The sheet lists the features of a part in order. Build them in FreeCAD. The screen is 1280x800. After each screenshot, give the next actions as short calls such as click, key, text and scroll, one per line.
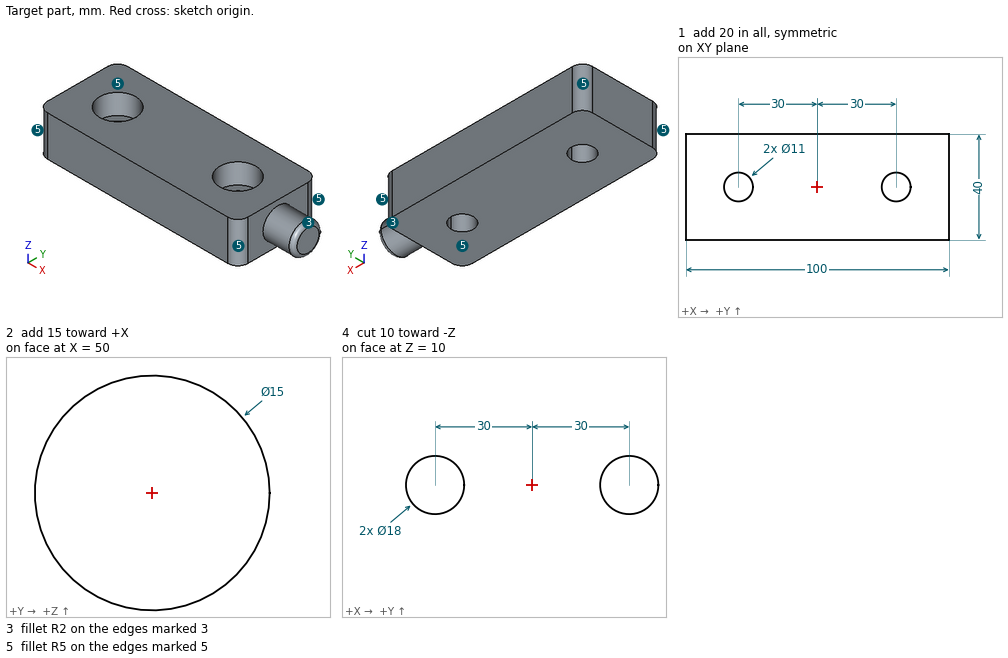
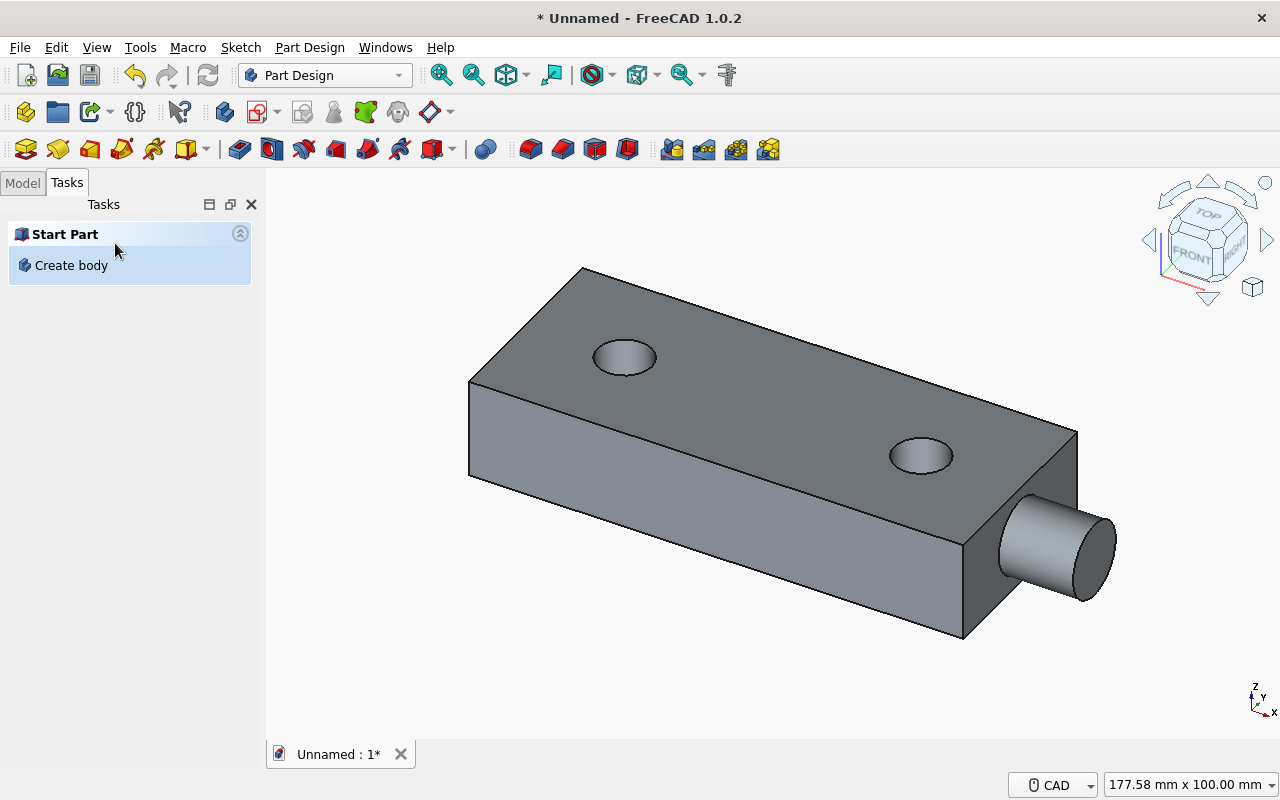
click(1073, 580)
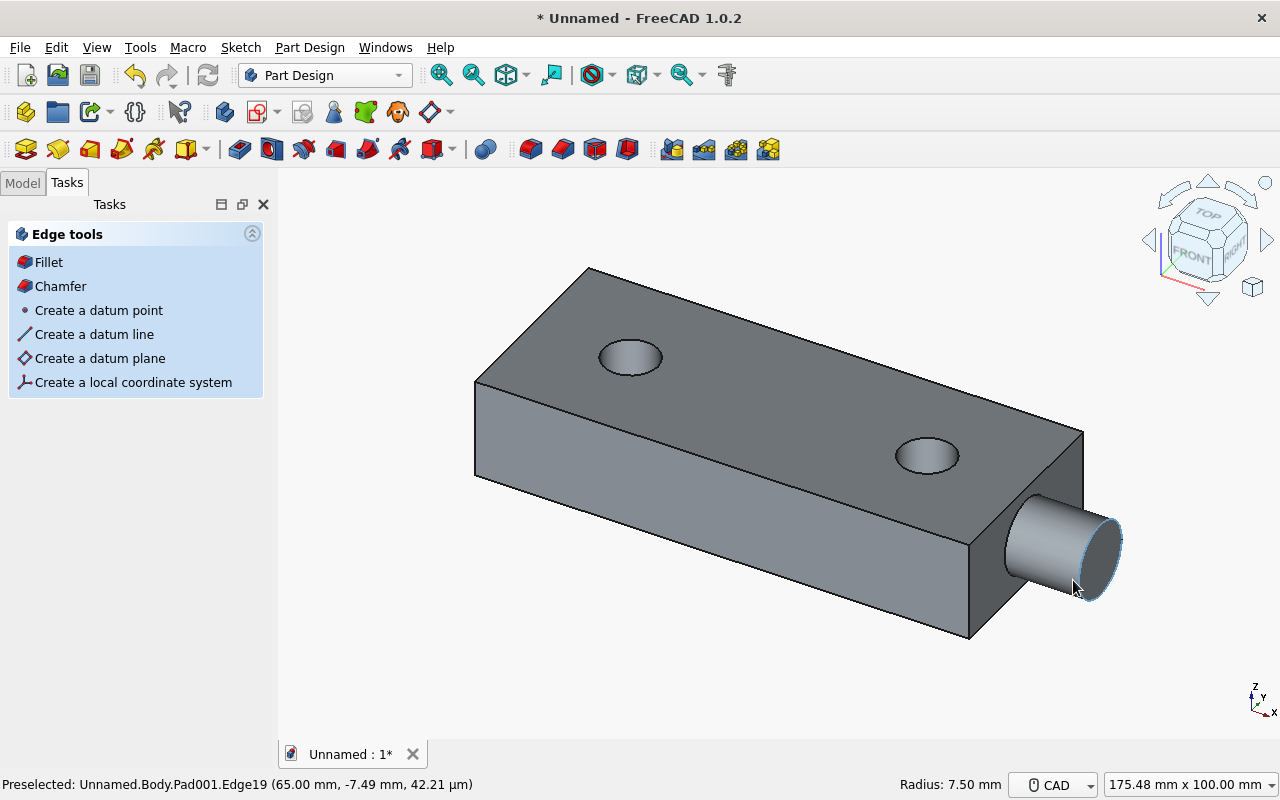
click(532, 150)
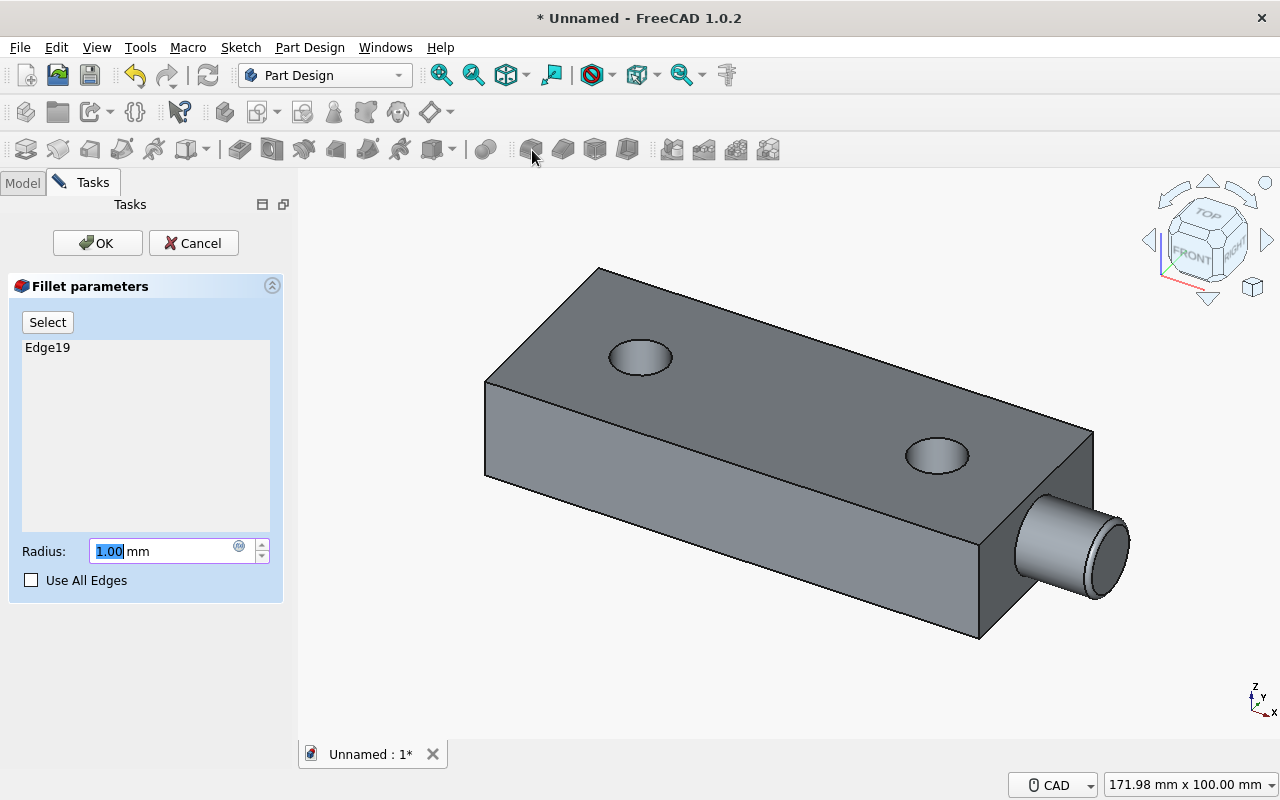
text(2)
key(Tab)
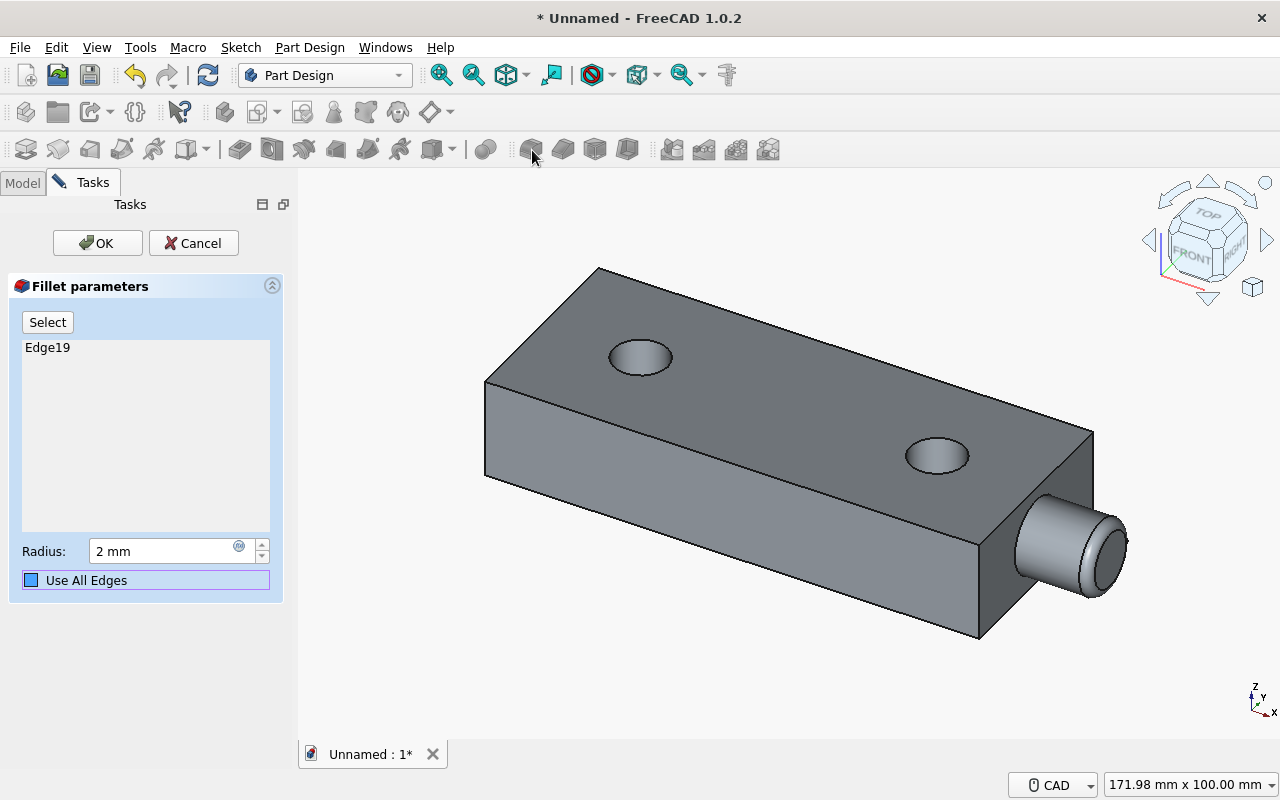
click(98, 243)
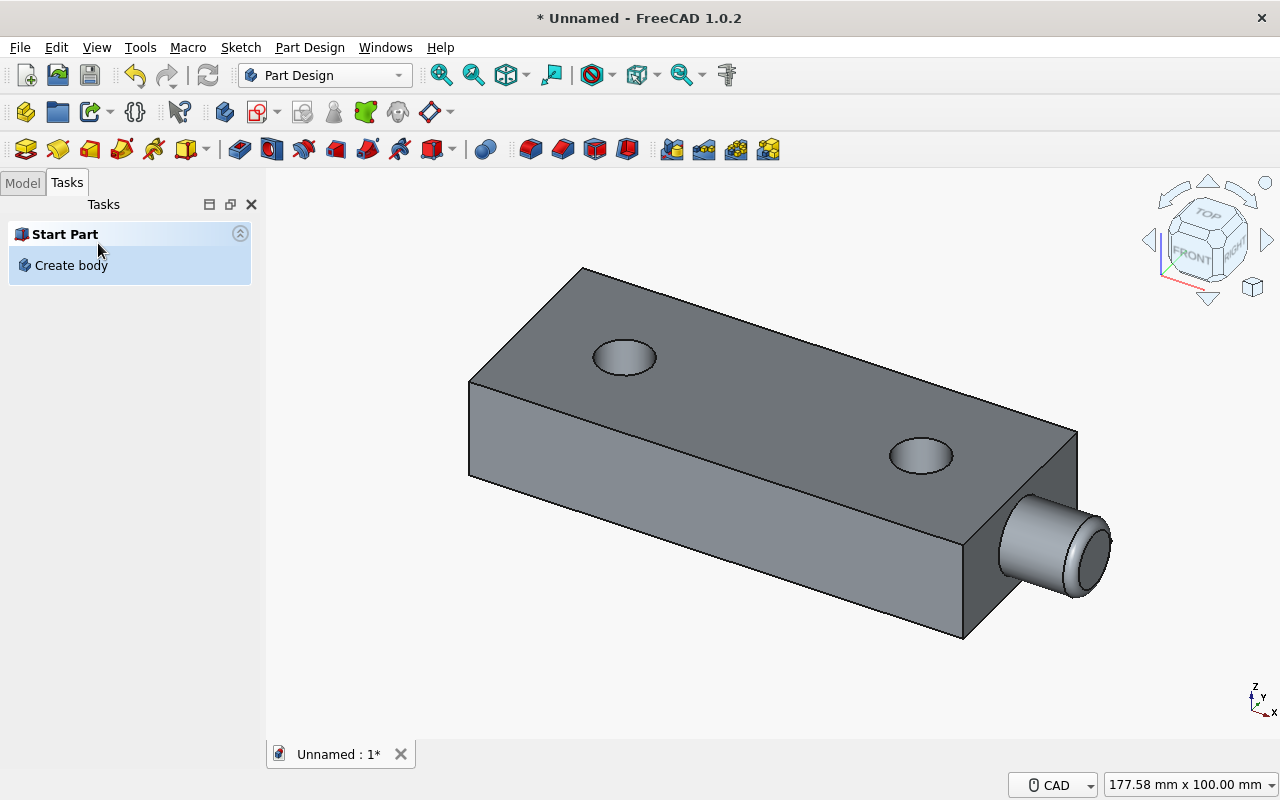
click(773, 406)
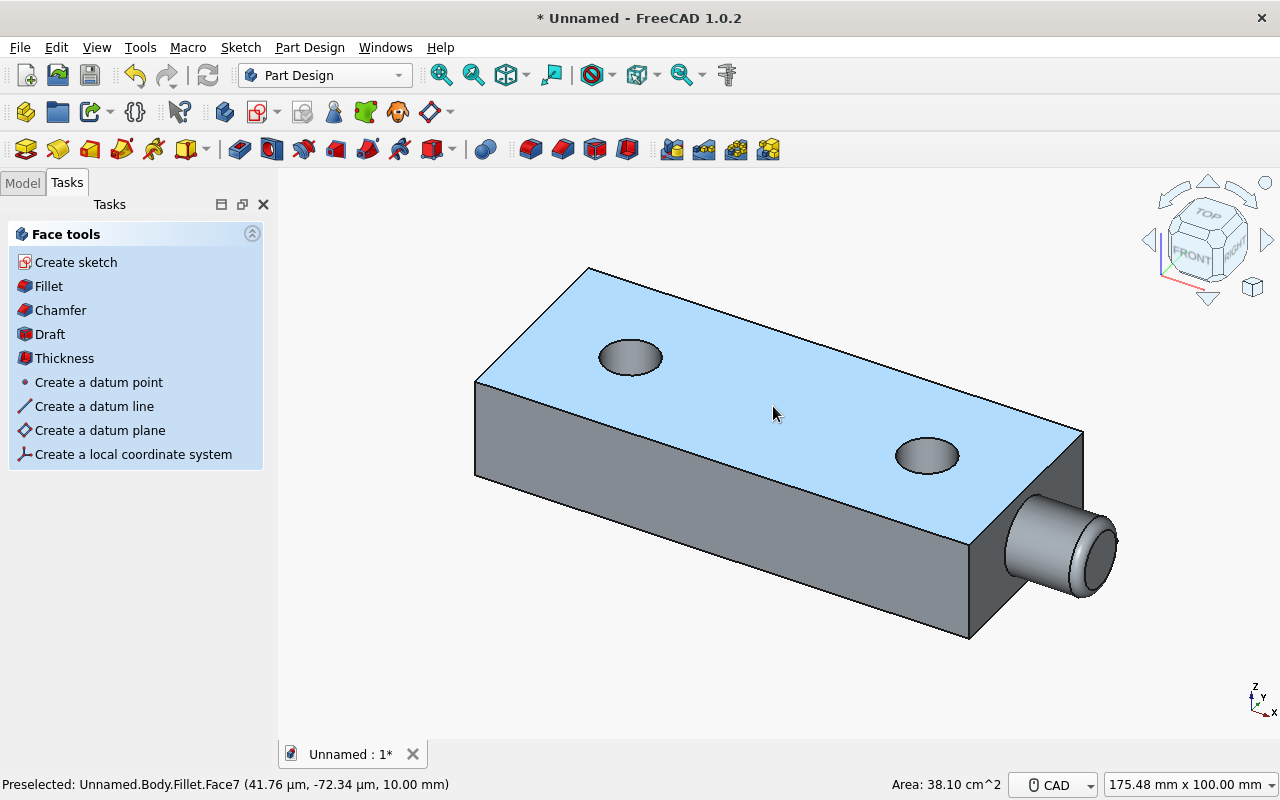
click(258, 112)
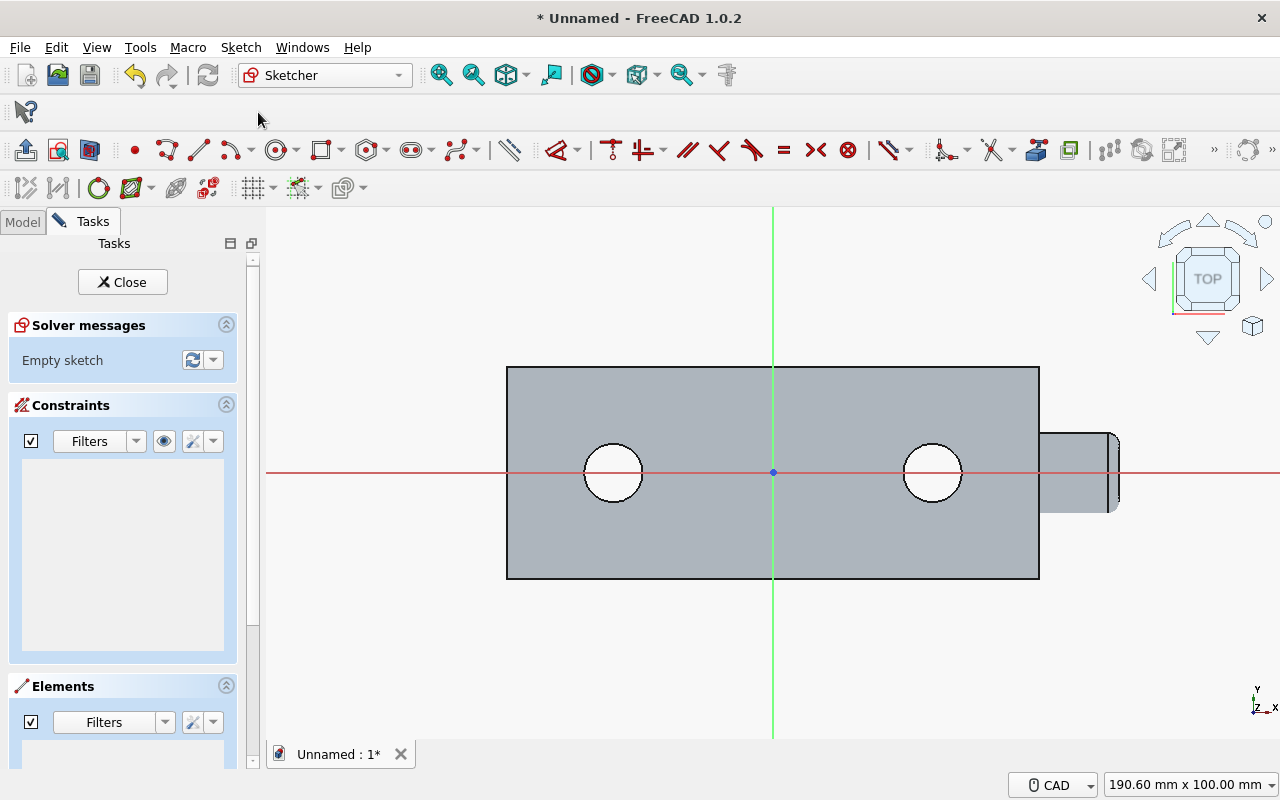
scroll(912, 473, up, 2)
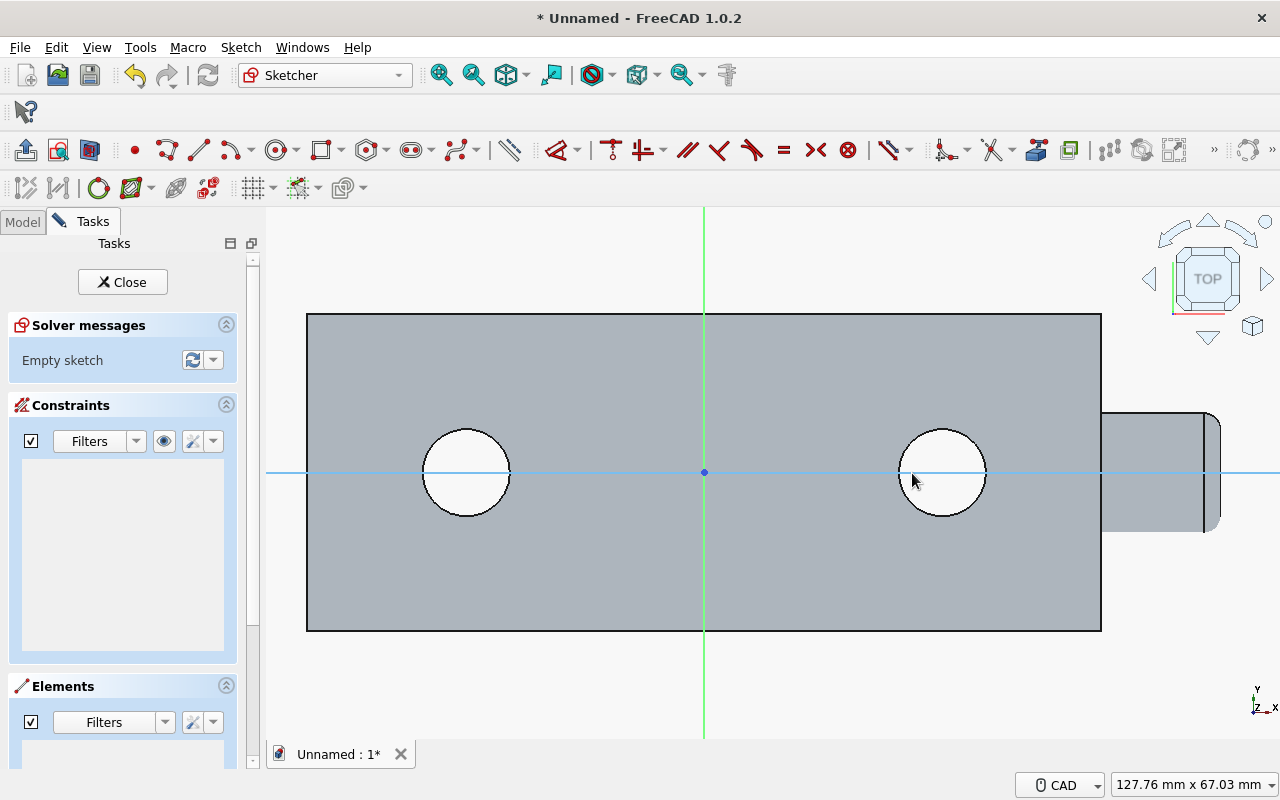
key(g)
key(c)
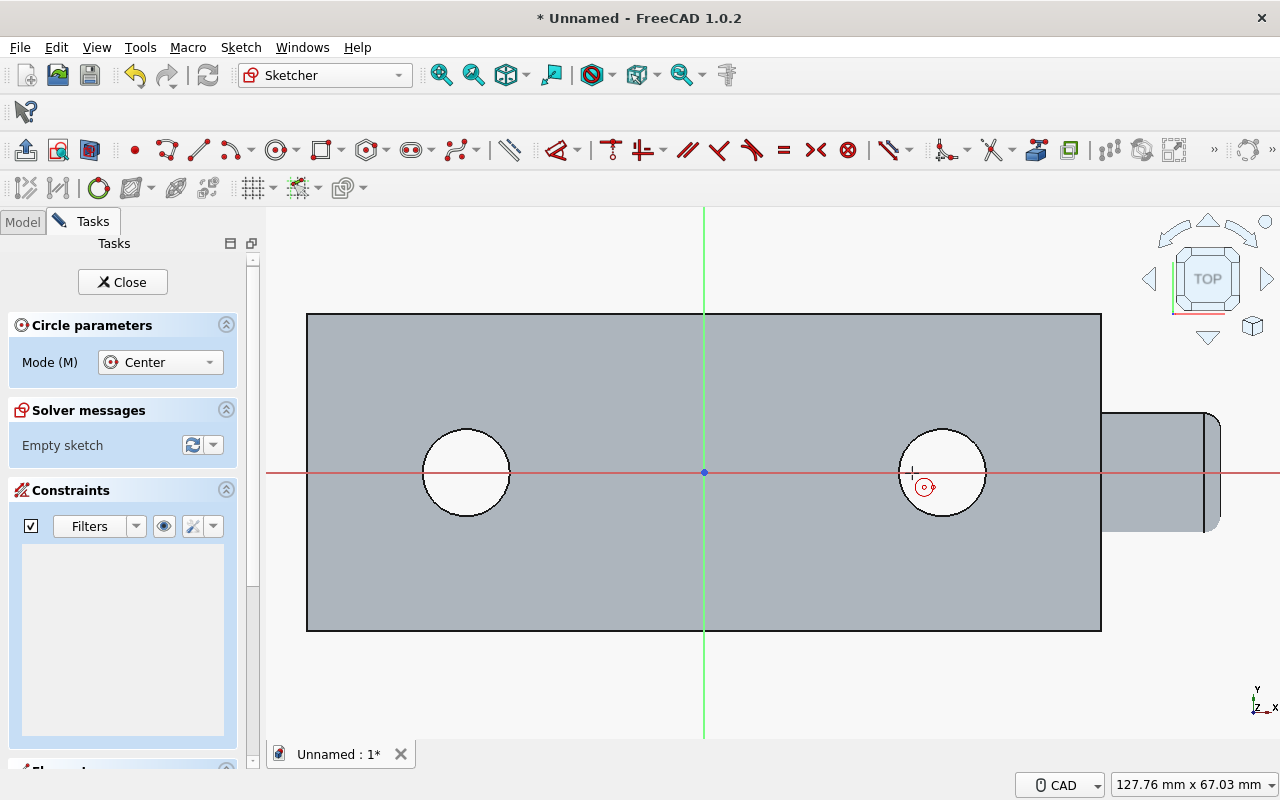
click(466, 473)
click(517, 422)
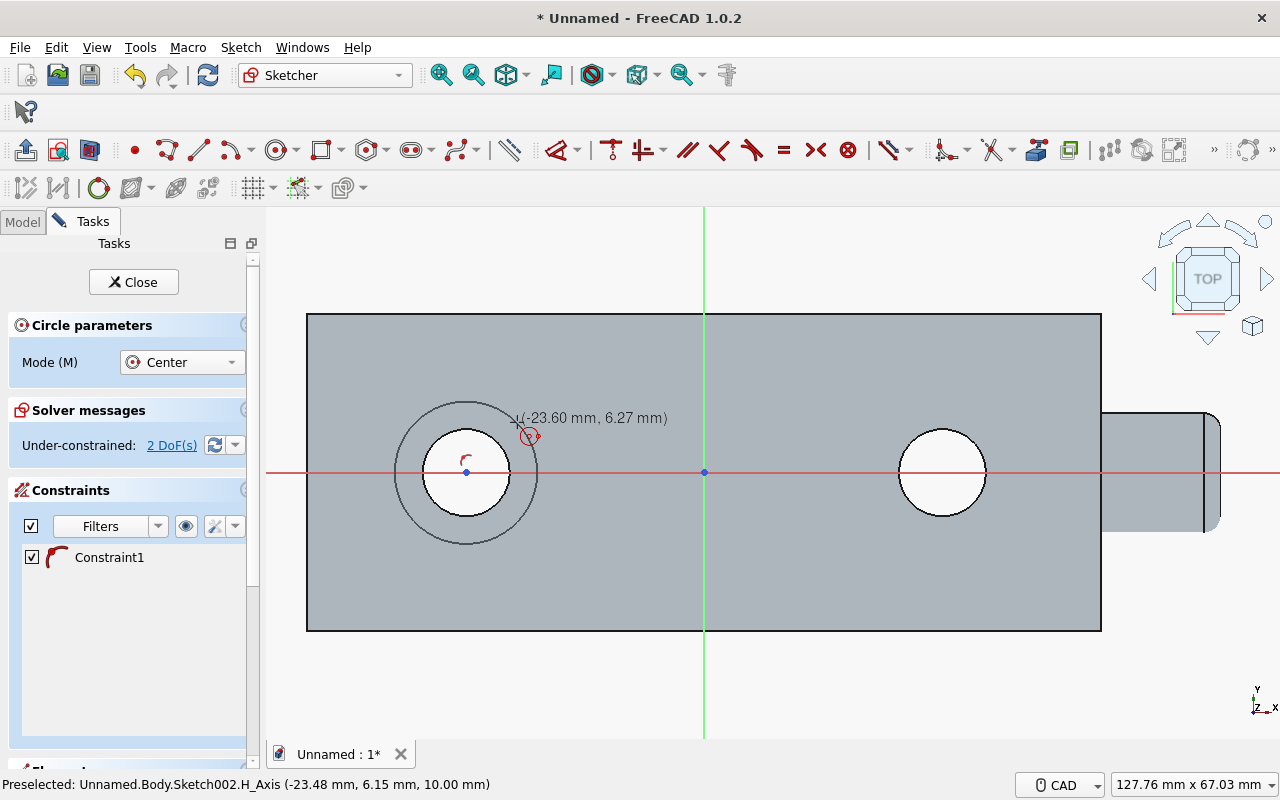
click(942, 473)
click(993, 422)
key(Escape)